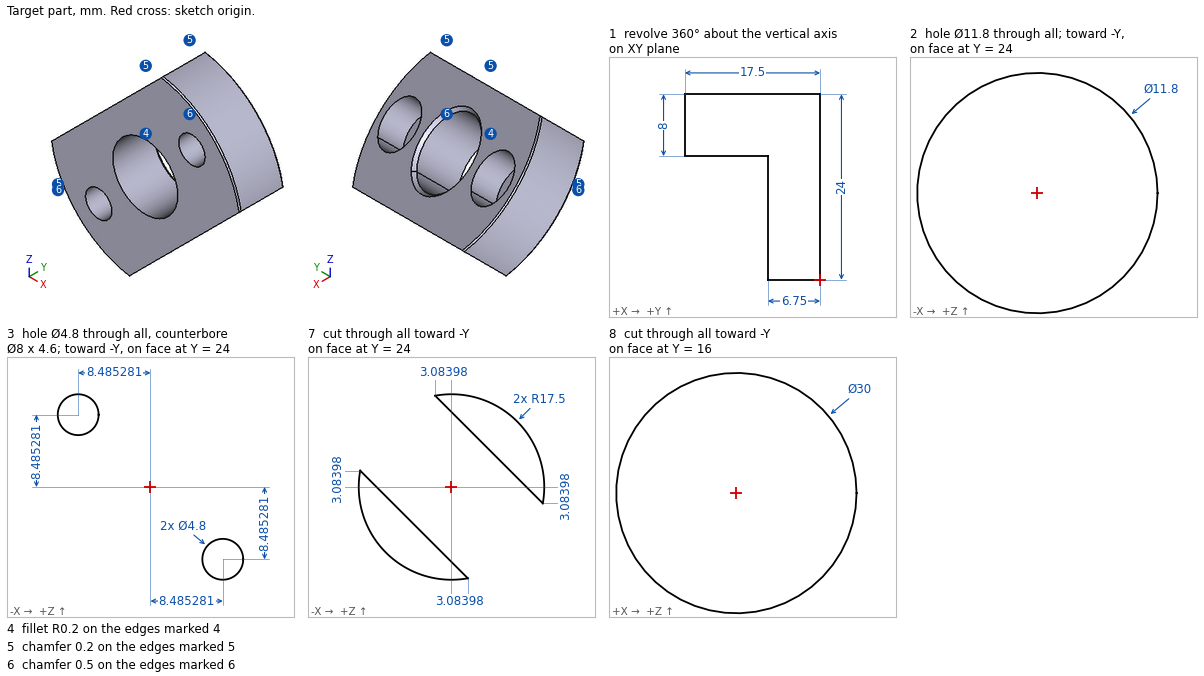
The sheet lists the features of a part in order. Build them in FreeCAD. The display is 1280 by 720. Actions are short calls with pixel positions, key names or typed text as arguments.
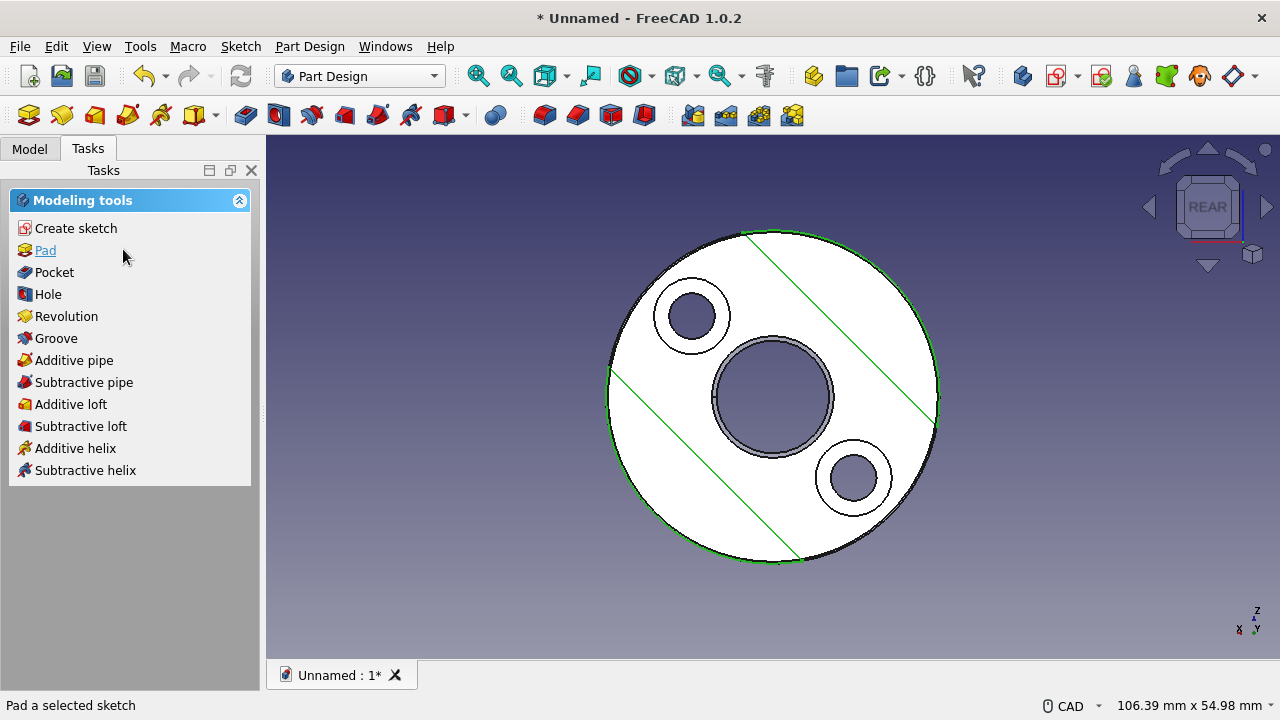
click(246, 116)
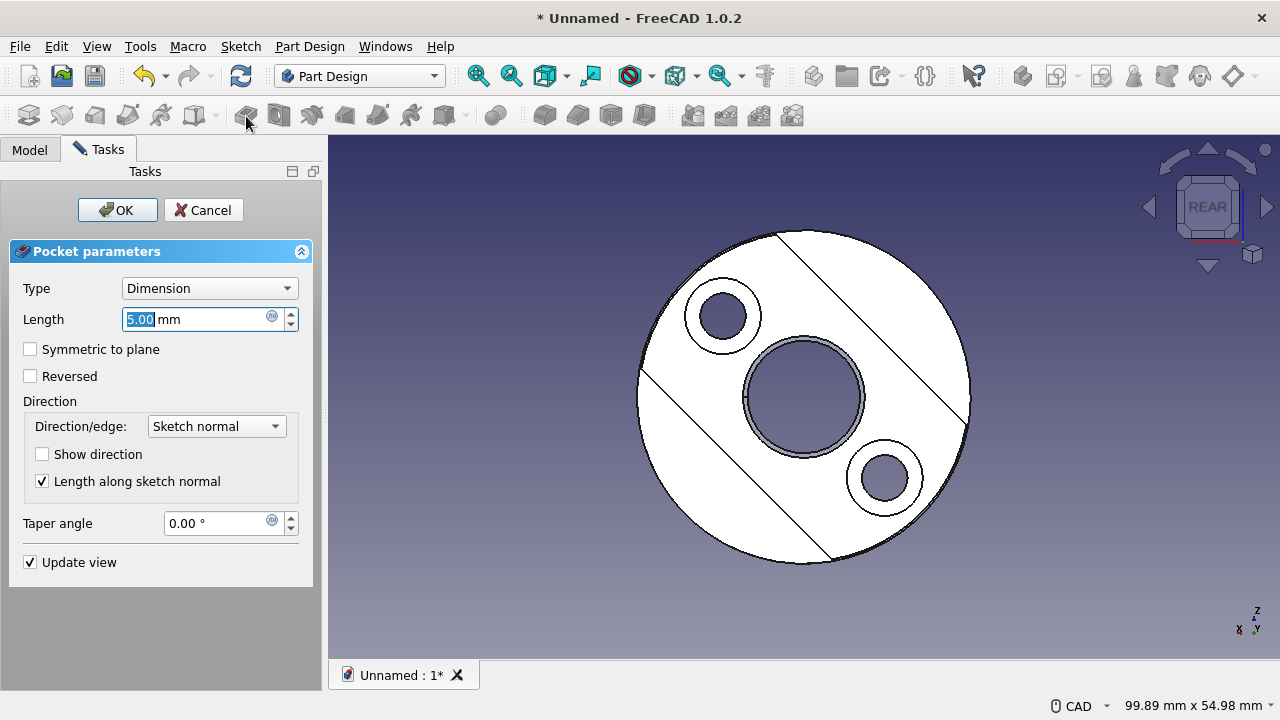
click(210, 288)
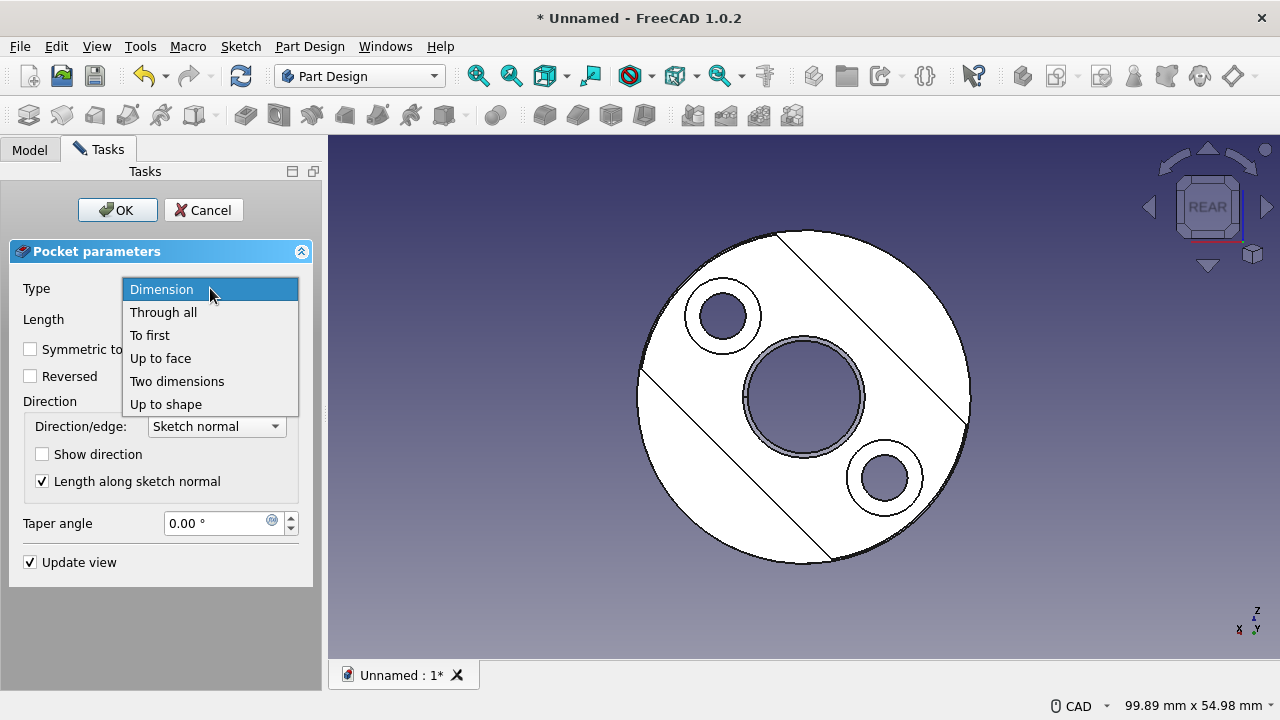
click(208, 312)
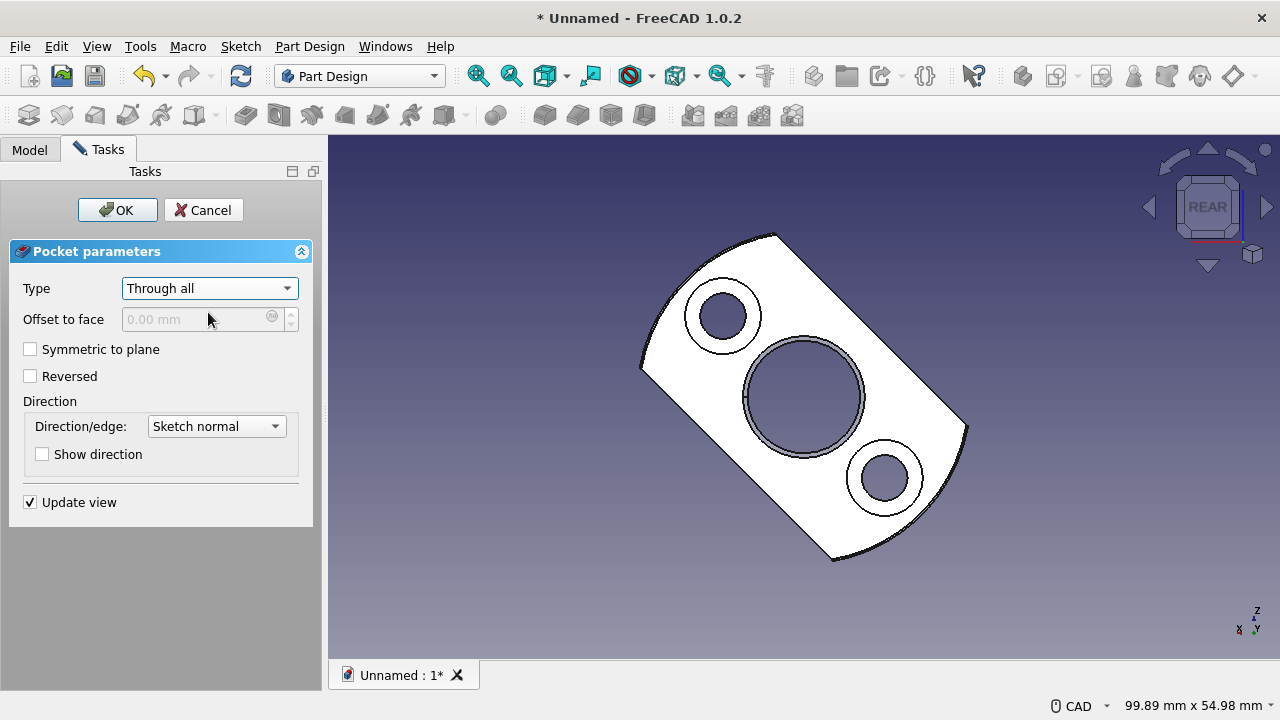
click(118, 210)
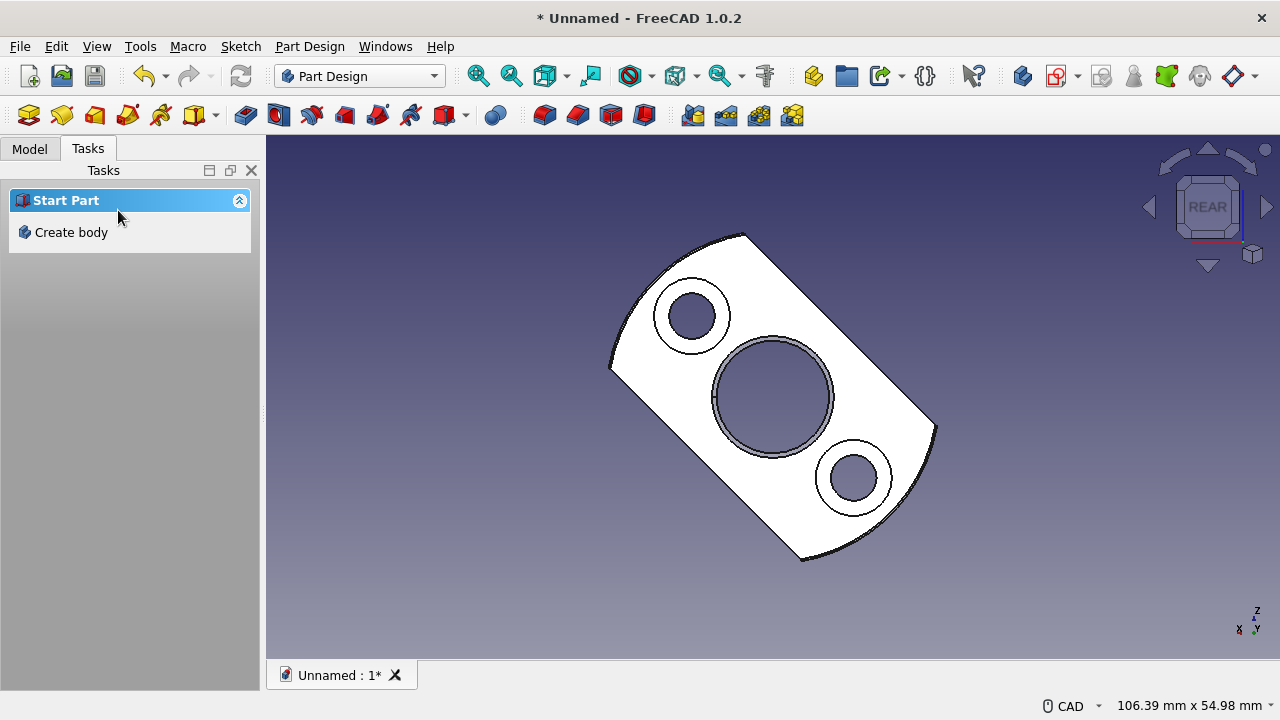
key(0)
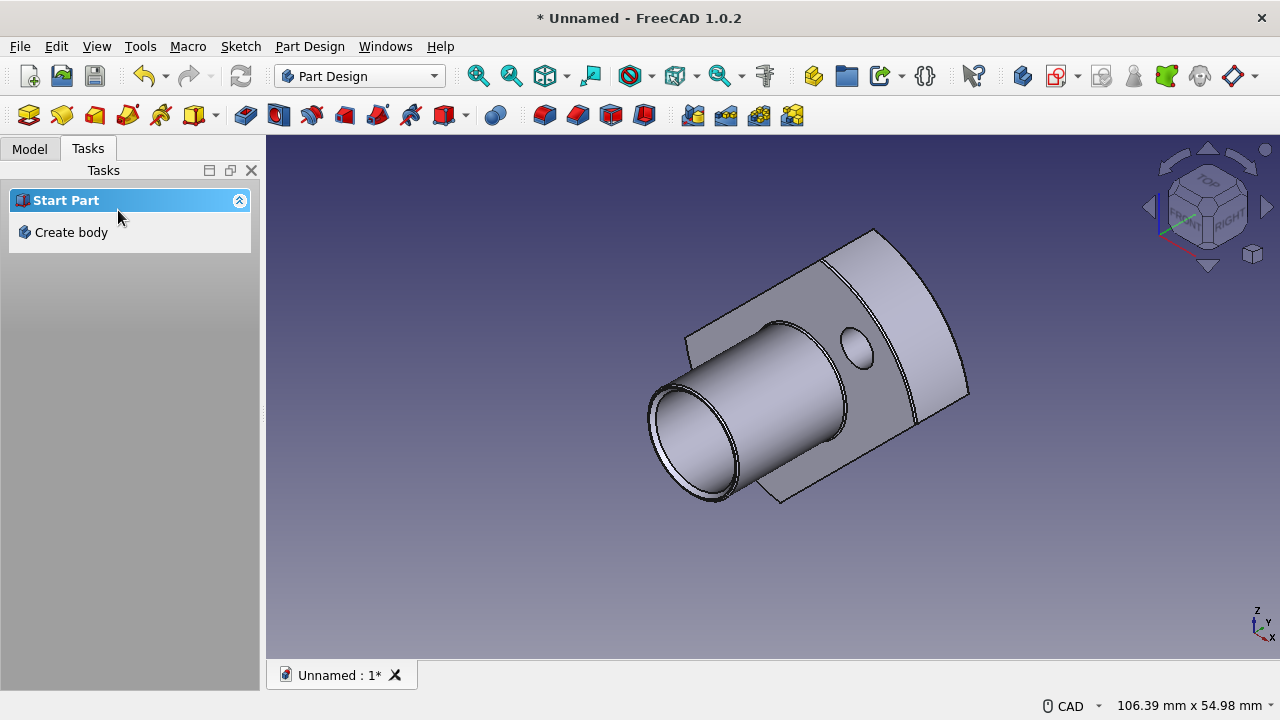
click(866, 418)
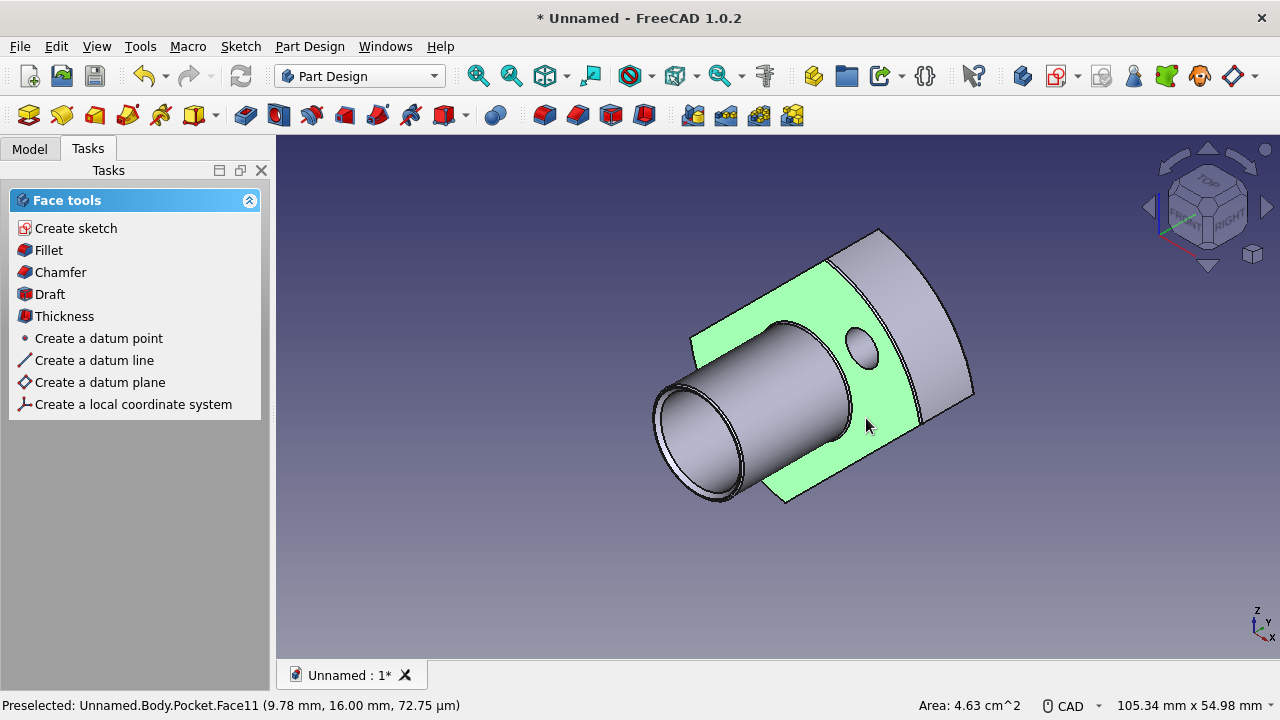
click(1056, 76)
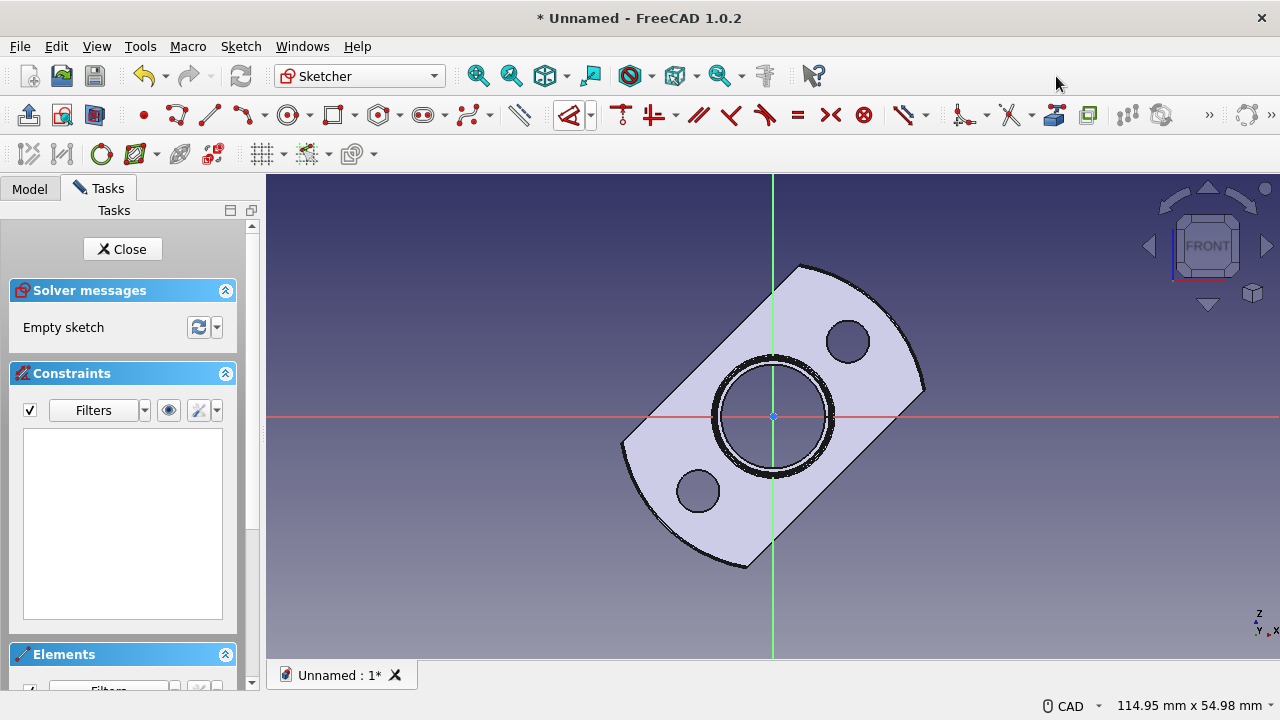
click(288, 116)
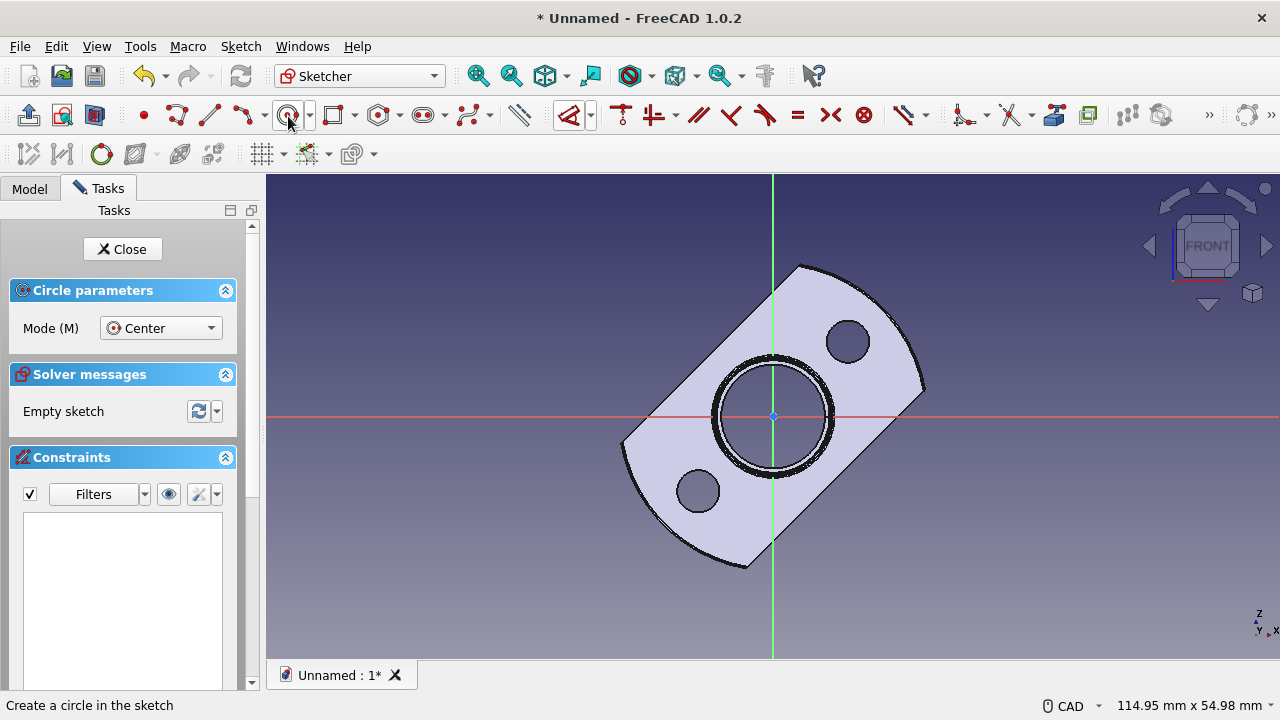
click(773, 417)
move(867, 323)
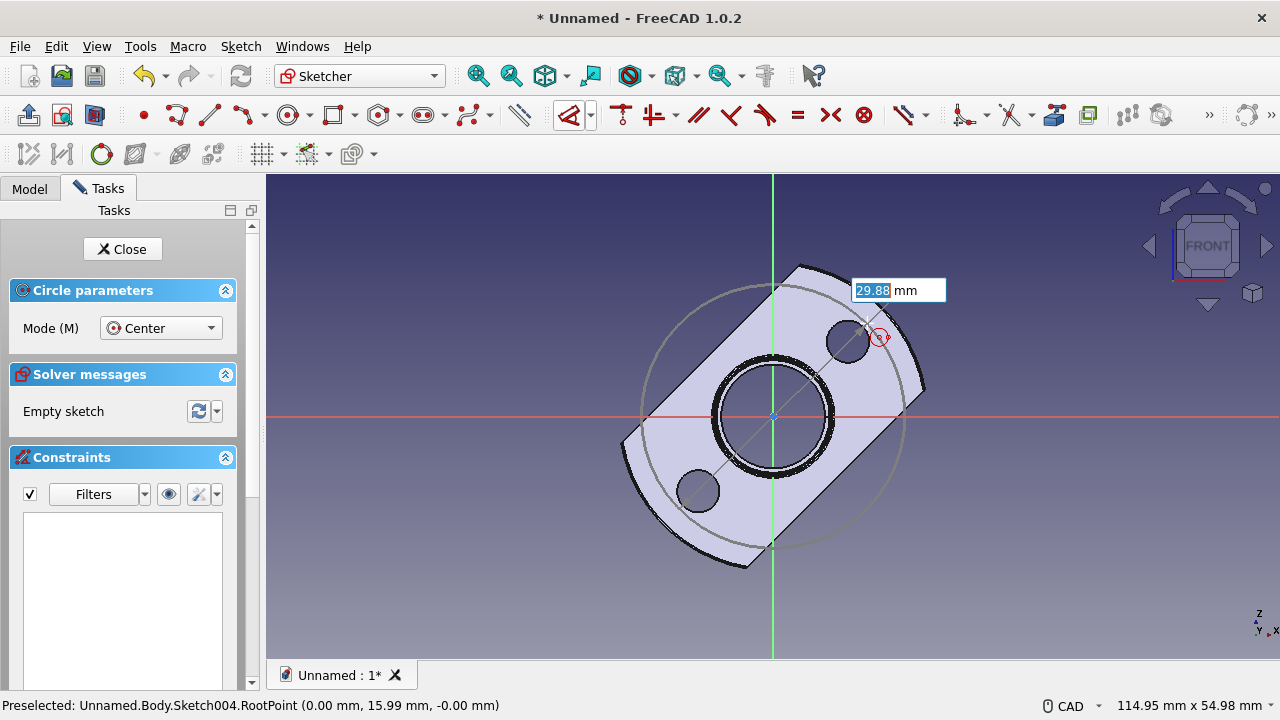
text(30)
key(Return)
key(Escape)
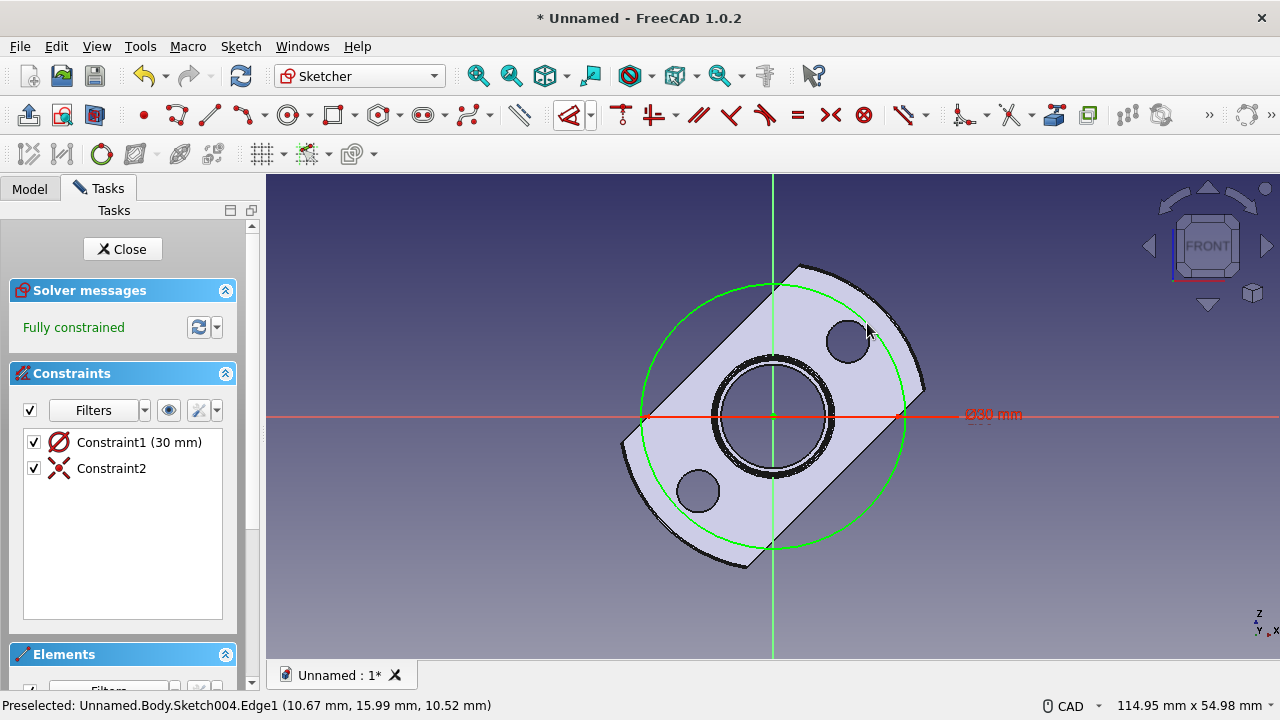
click(123, 249)